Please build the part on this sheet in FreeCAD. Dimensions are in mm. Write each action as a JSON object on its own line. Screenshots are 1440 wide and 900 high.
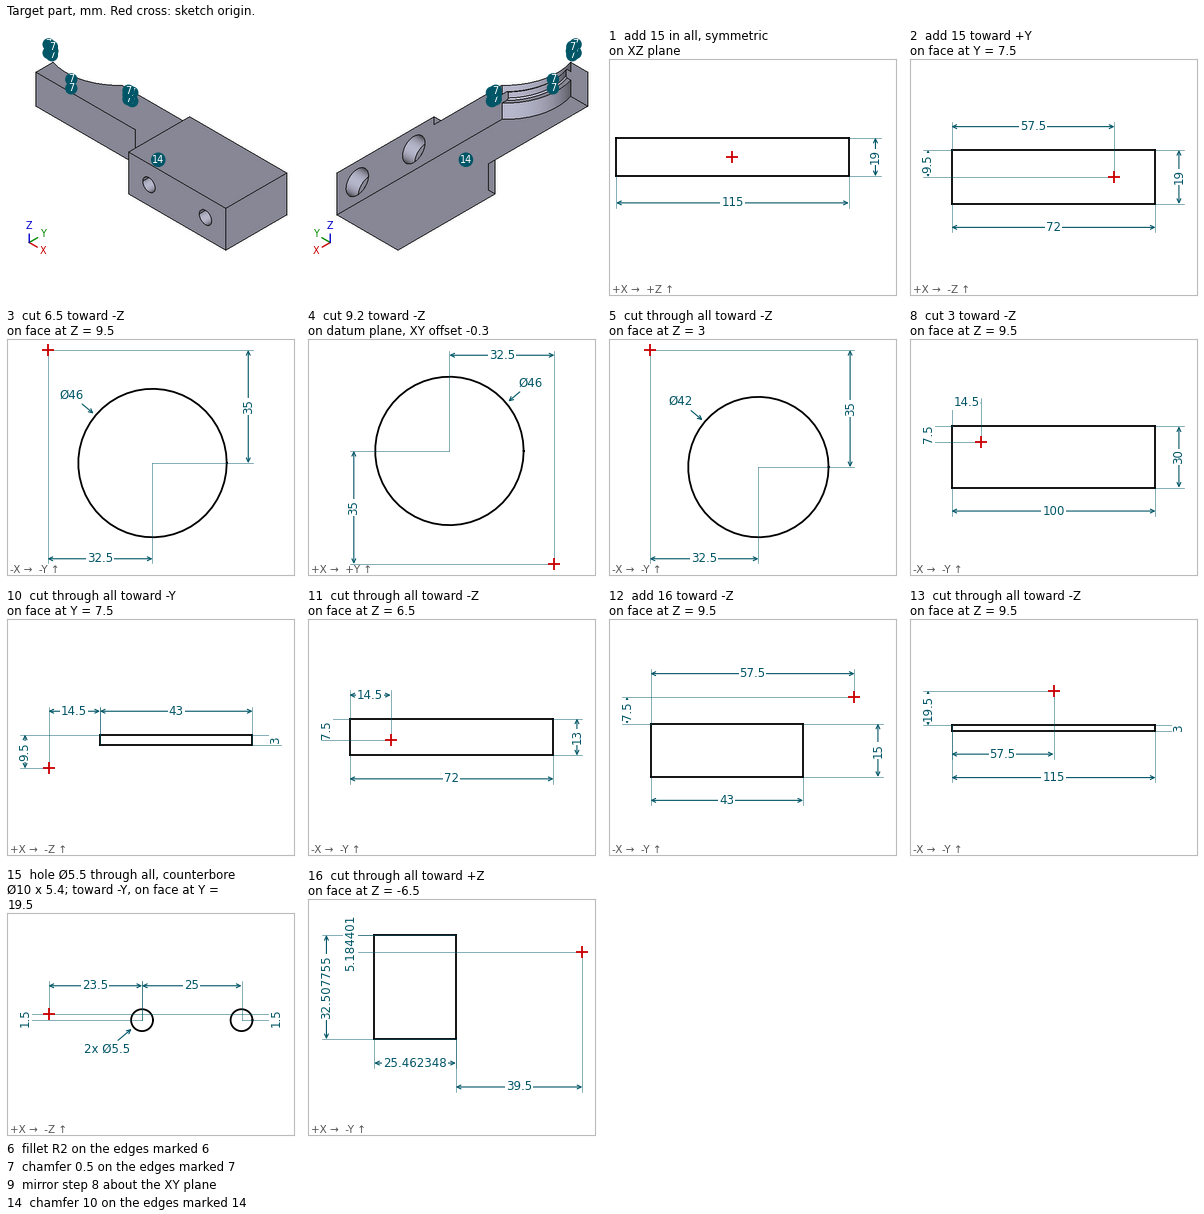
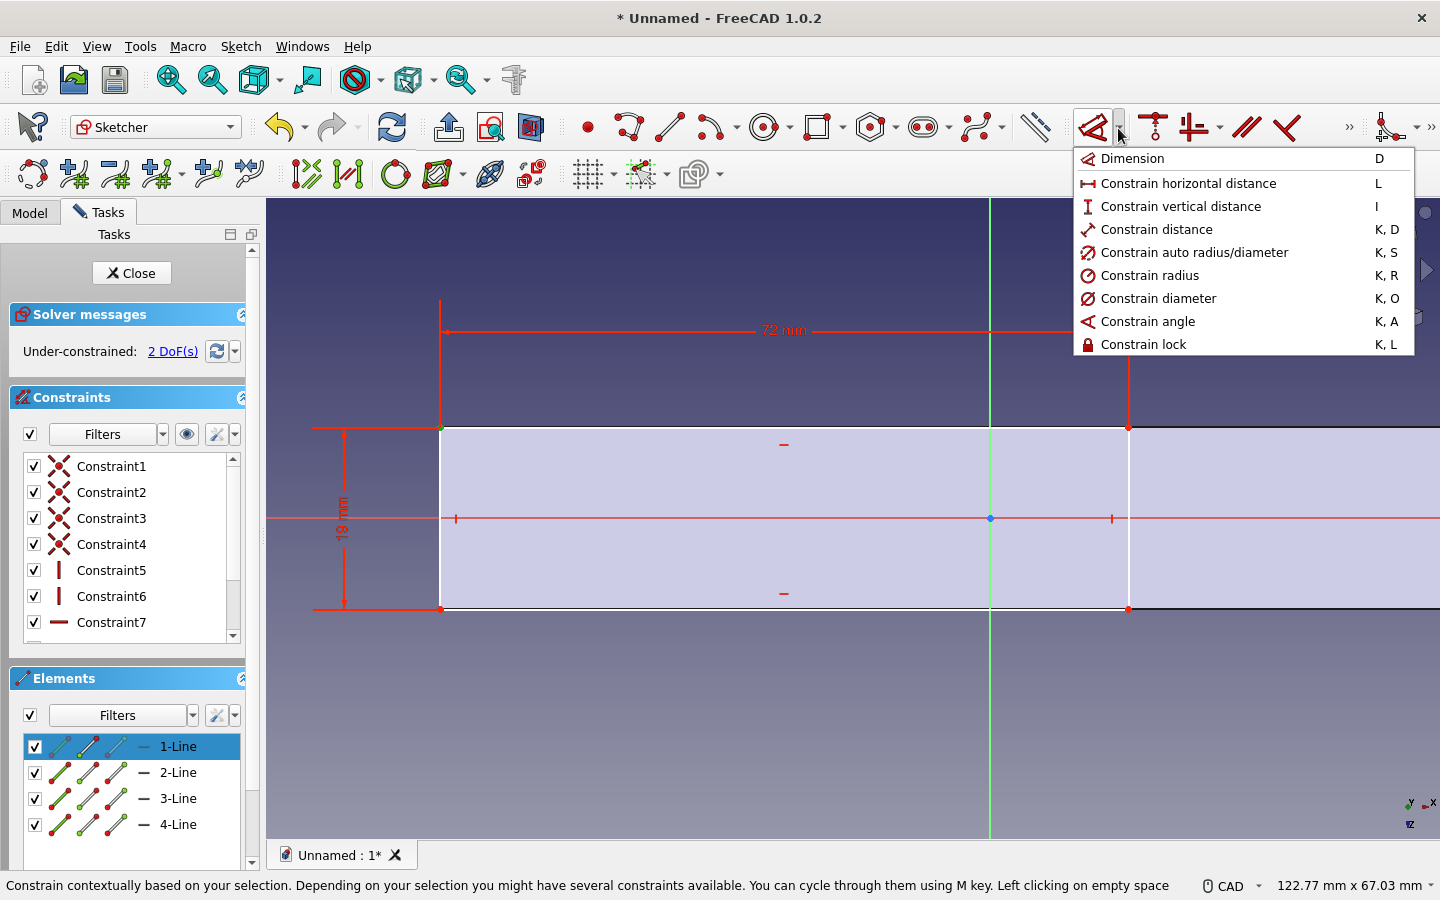
{"action": "left_click", "coordinate": [1244, 206]}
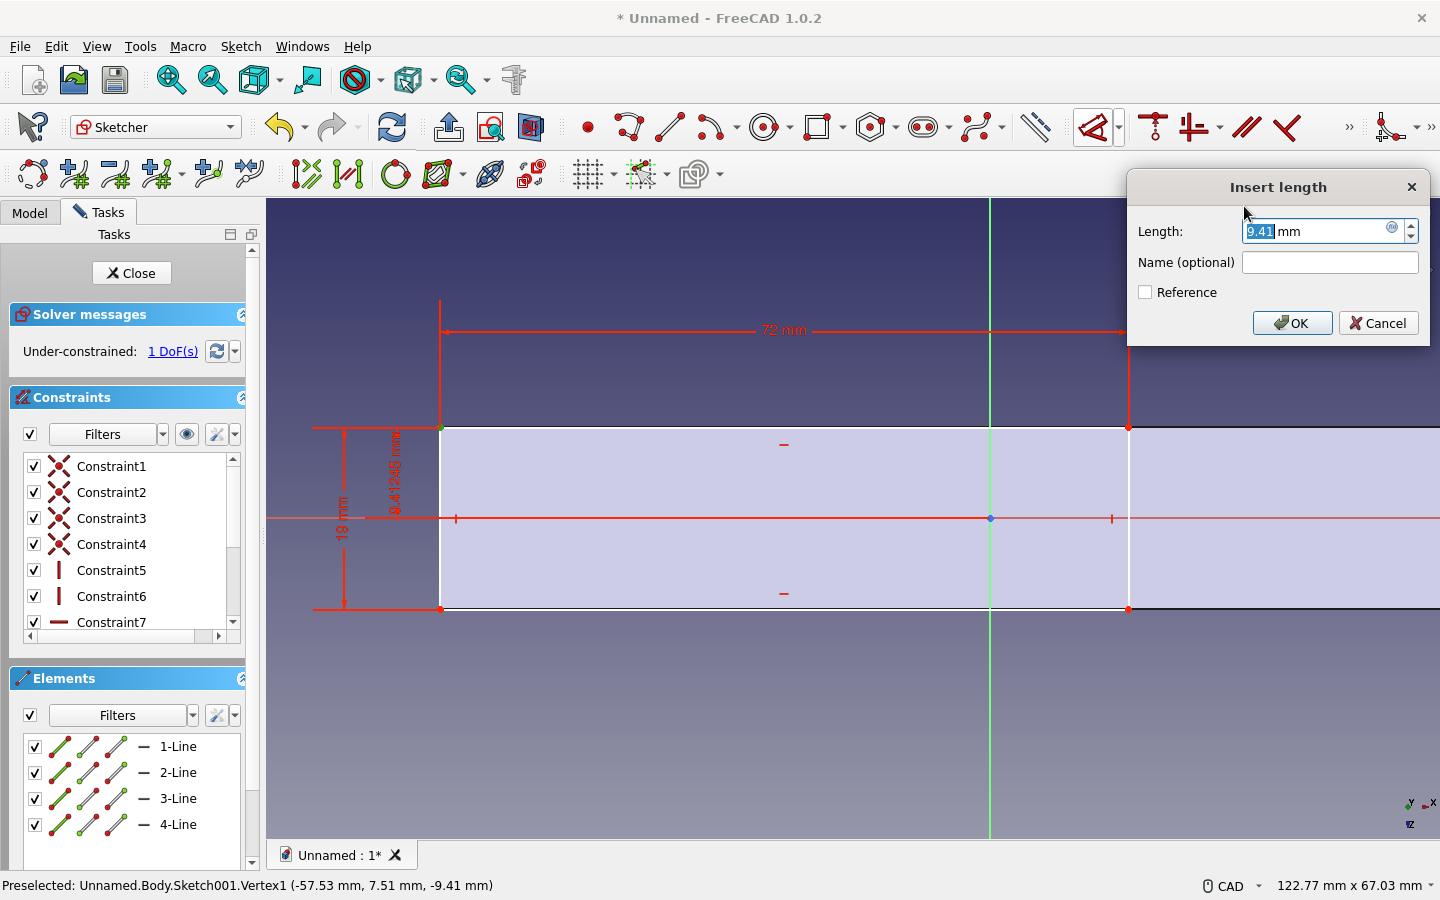
{"action": "type", "text": "9.5"}
{"action": "key", "text": "Return"}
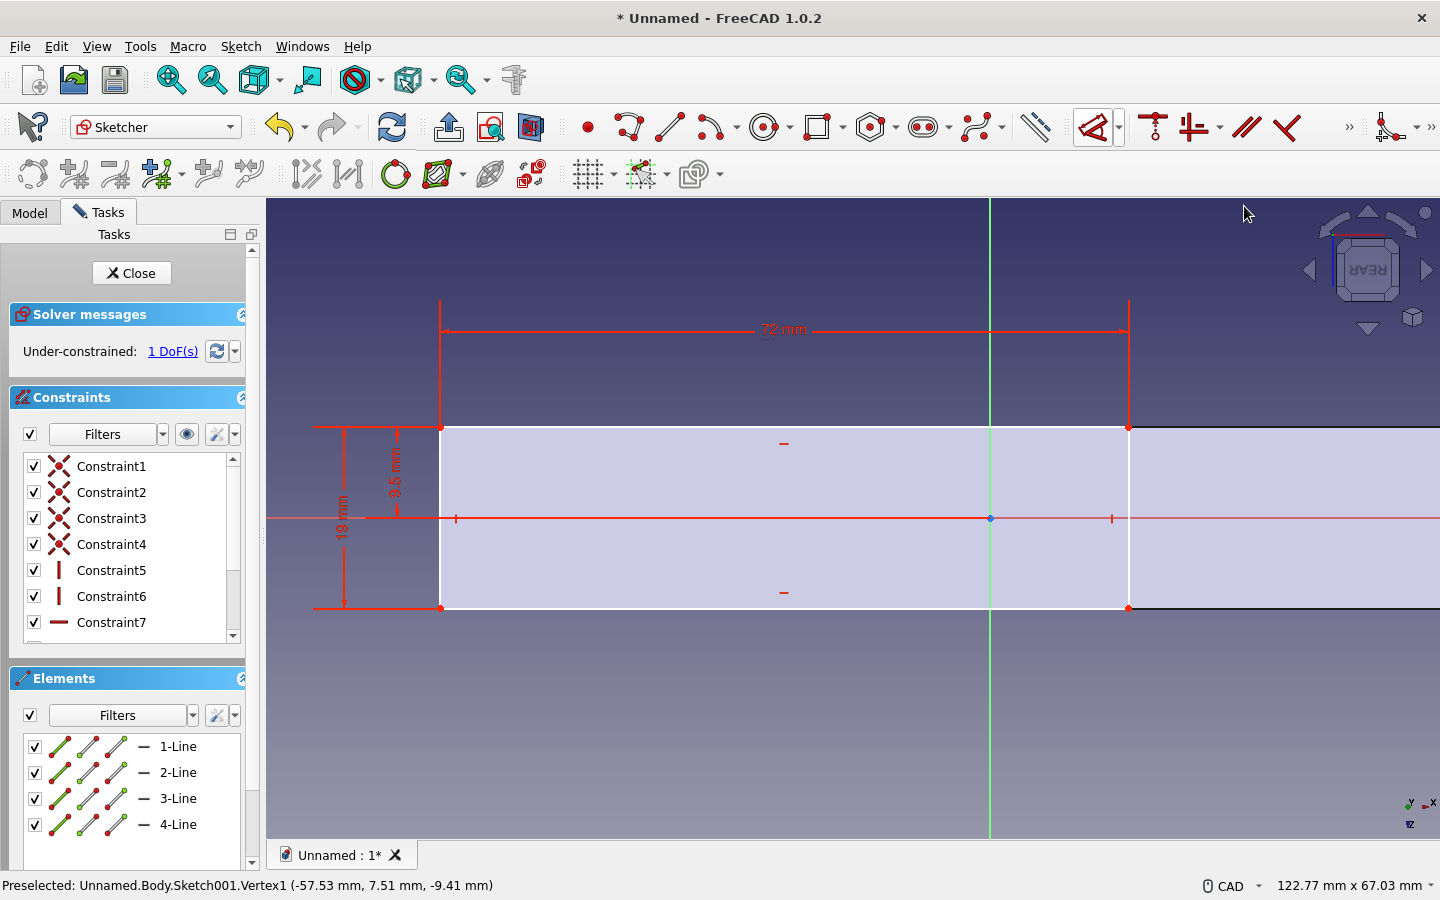
{"action": "left_click", "coordinate": [440, 427]}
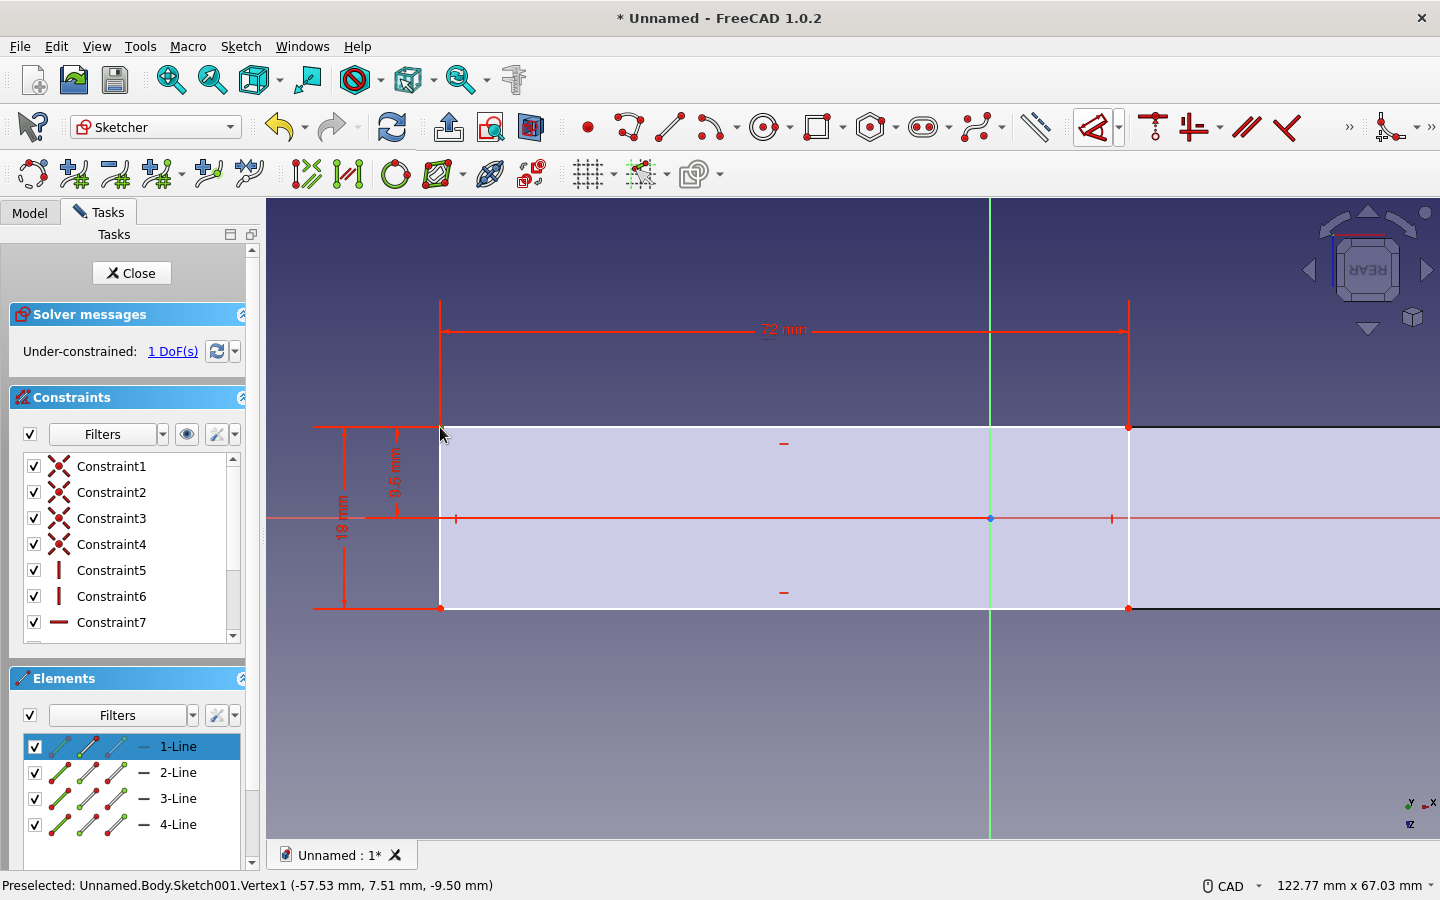
{"action": "key", "text": "l"}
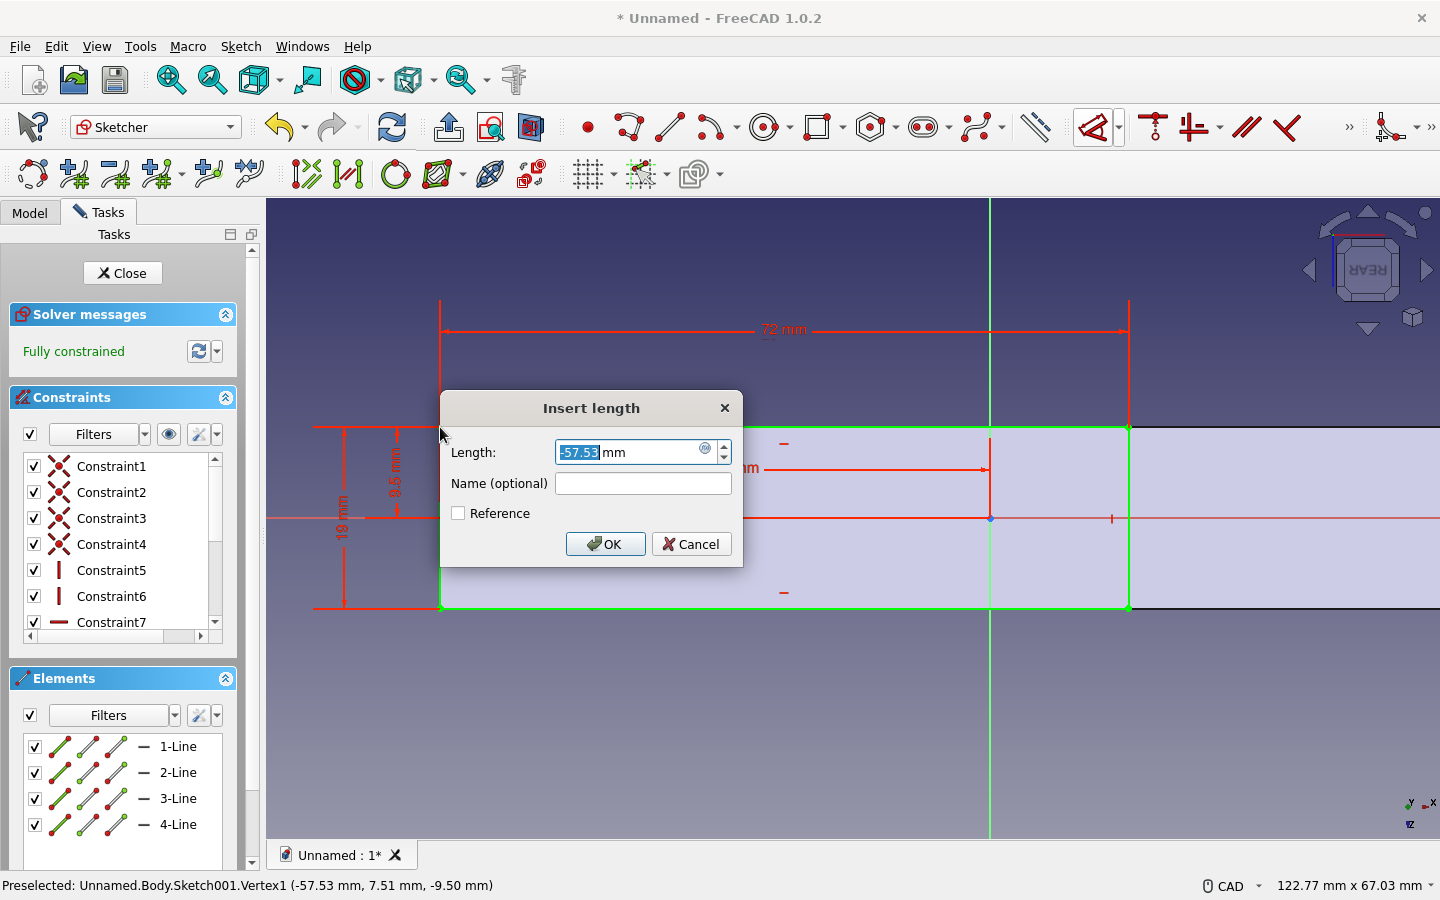
{"action": "type", "text": "-57.5"}
{"action": "key", "text": "Return"}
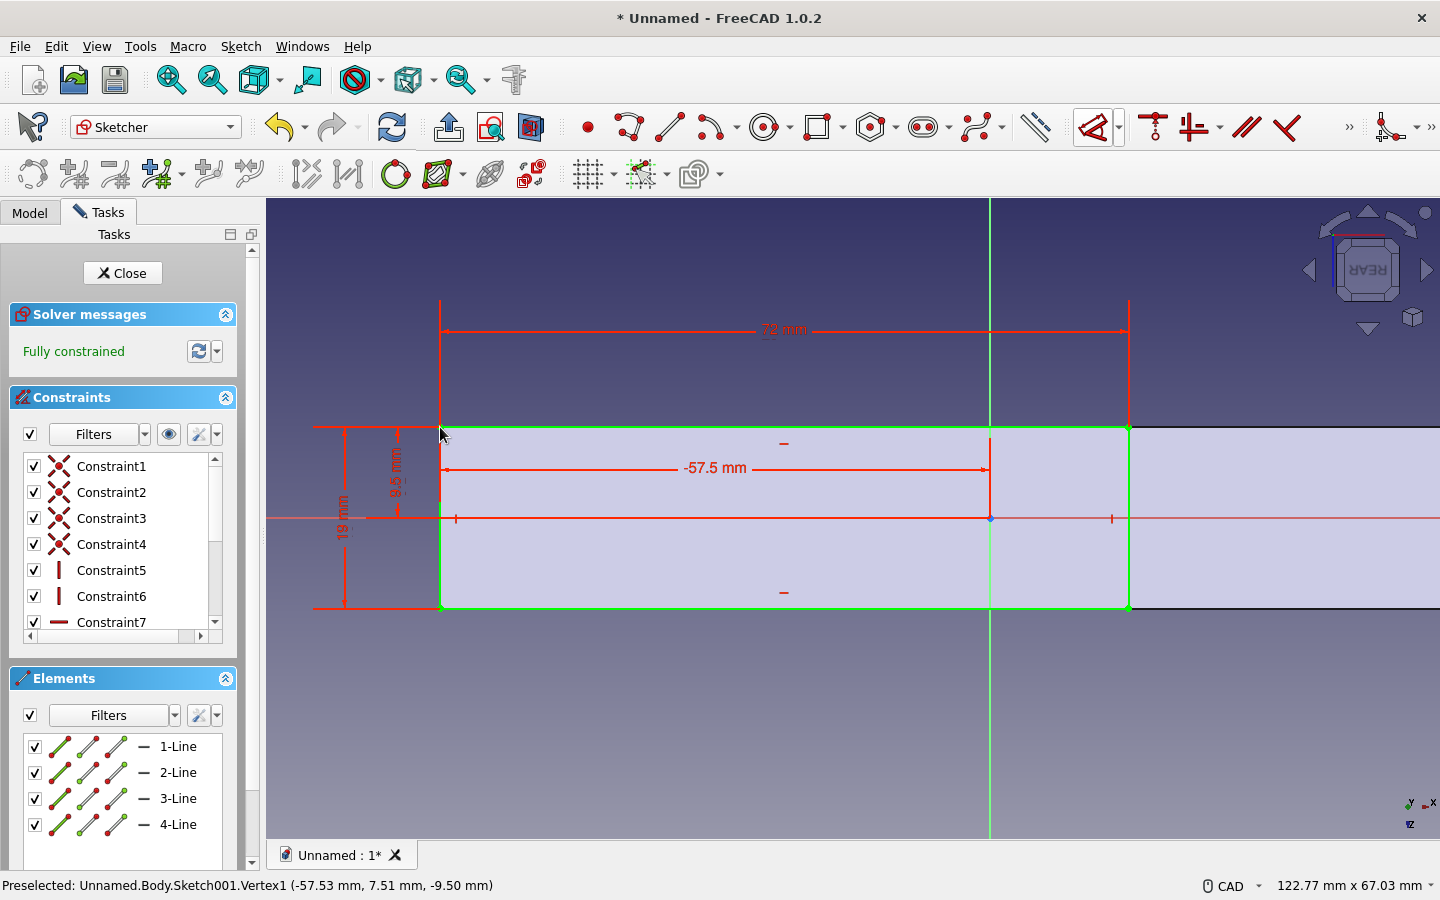
{"action": "left_click", "coordinate": [123, 273]}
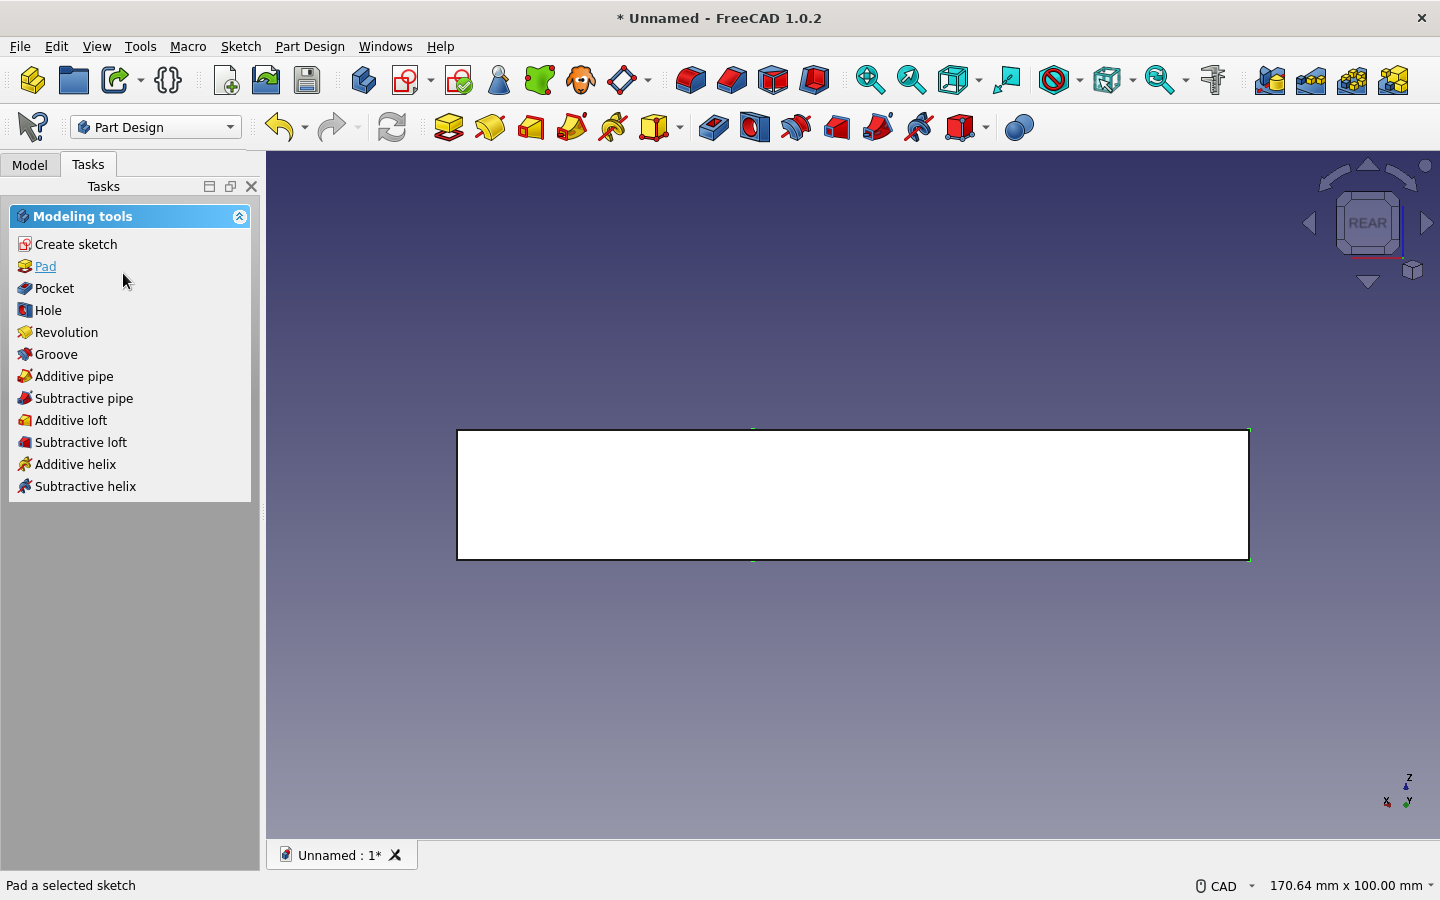
{"action": "left_click", "coordinate": [449, 128]}